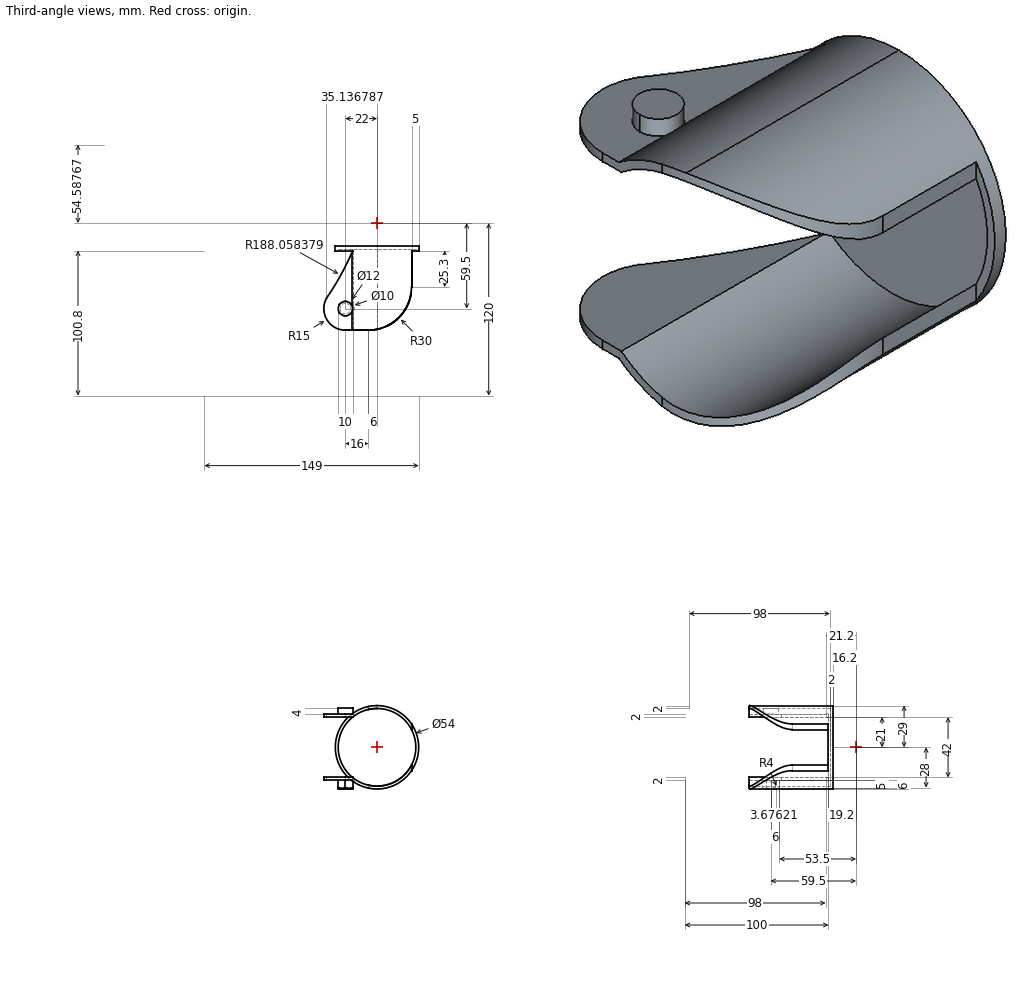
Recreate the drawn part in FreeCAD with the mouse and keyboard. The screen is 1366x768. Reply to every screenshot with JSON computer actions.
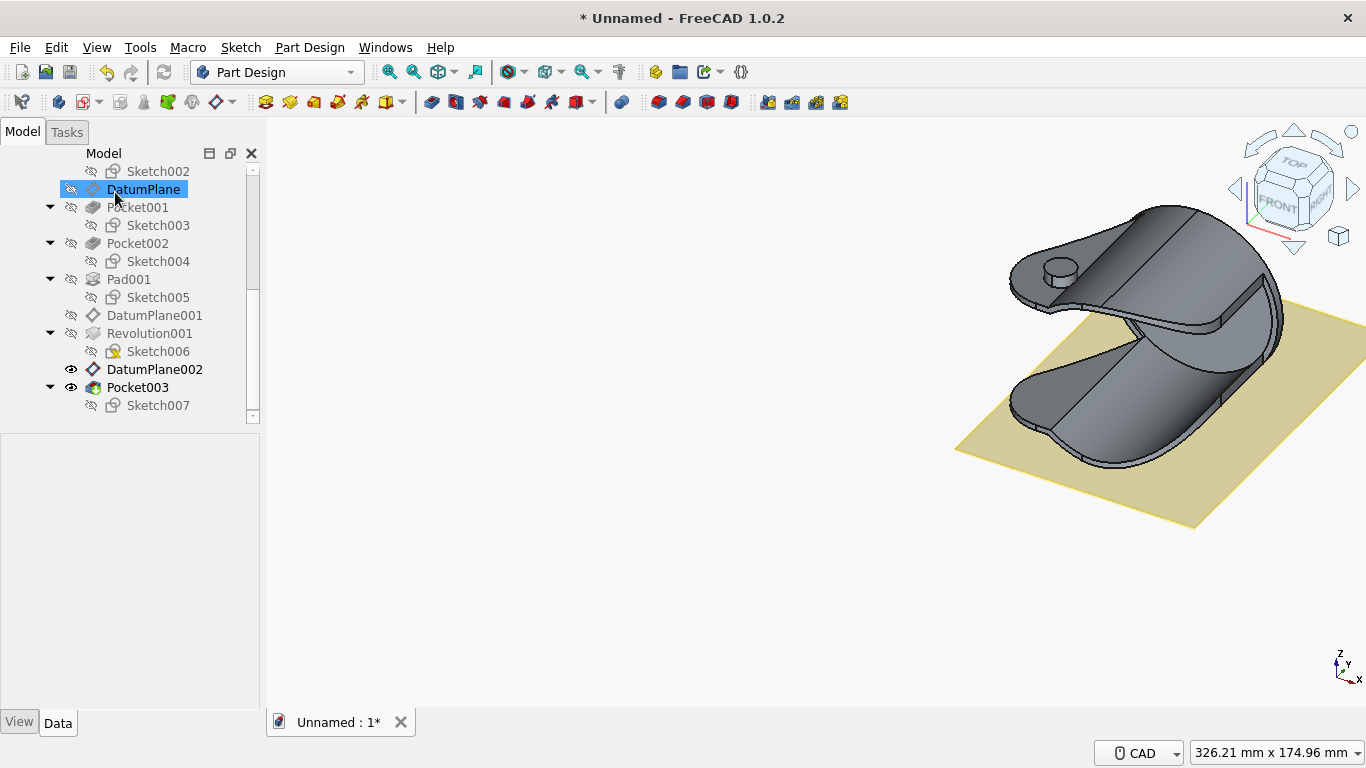
{"action": "left_click", "coordinate": [116, 369]}
{"action": "key", "text": "space"}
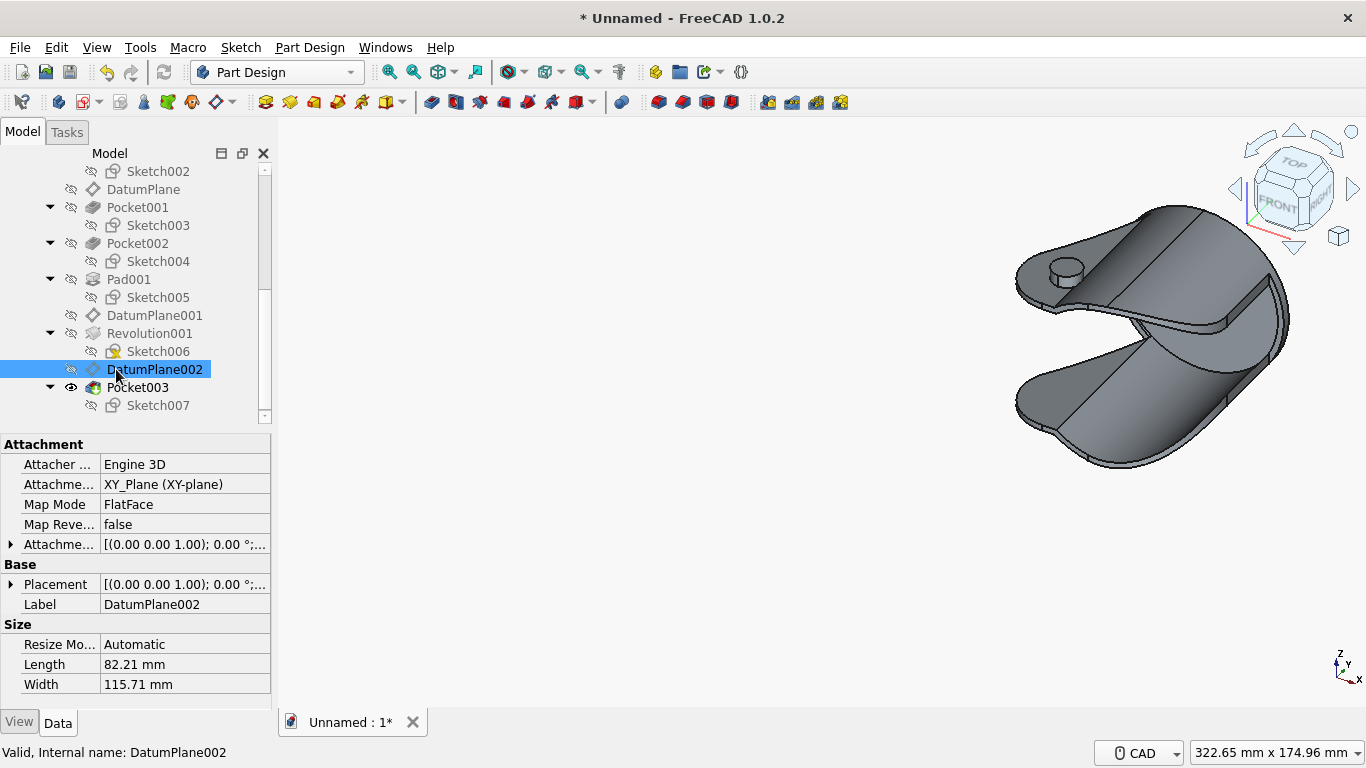
{"action": "key", "text": "0"}